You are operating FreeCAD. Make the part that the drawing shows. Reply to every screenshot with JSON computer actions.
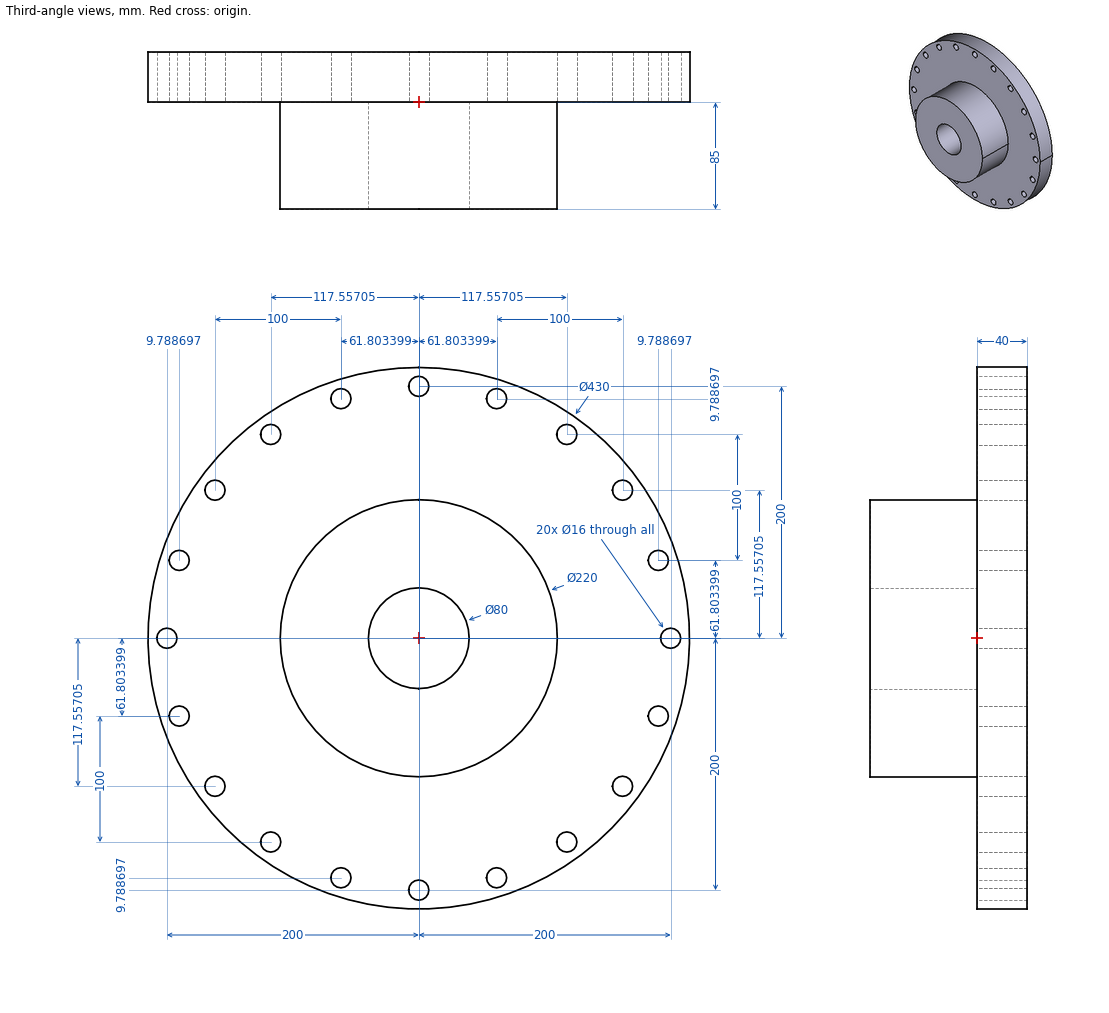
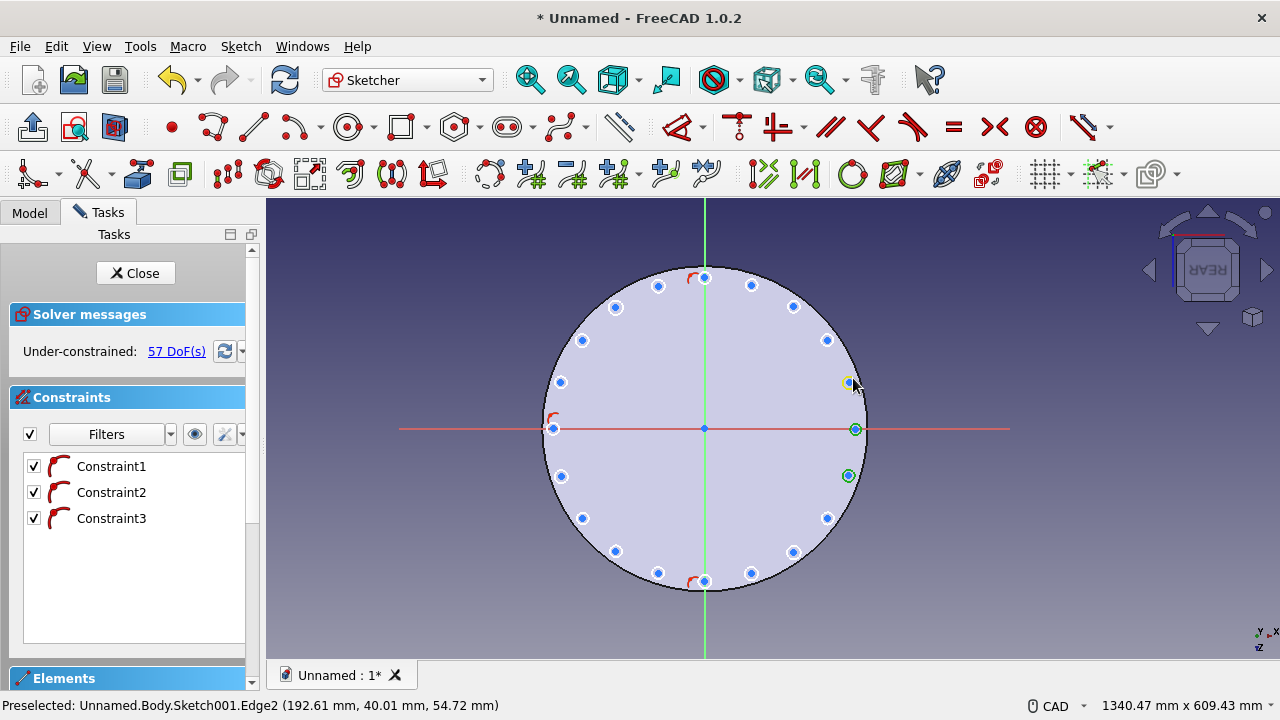
{"action": "scroll", "coordinate": [832, 514], "scroll_direction": "up", "scroll_amount": 5}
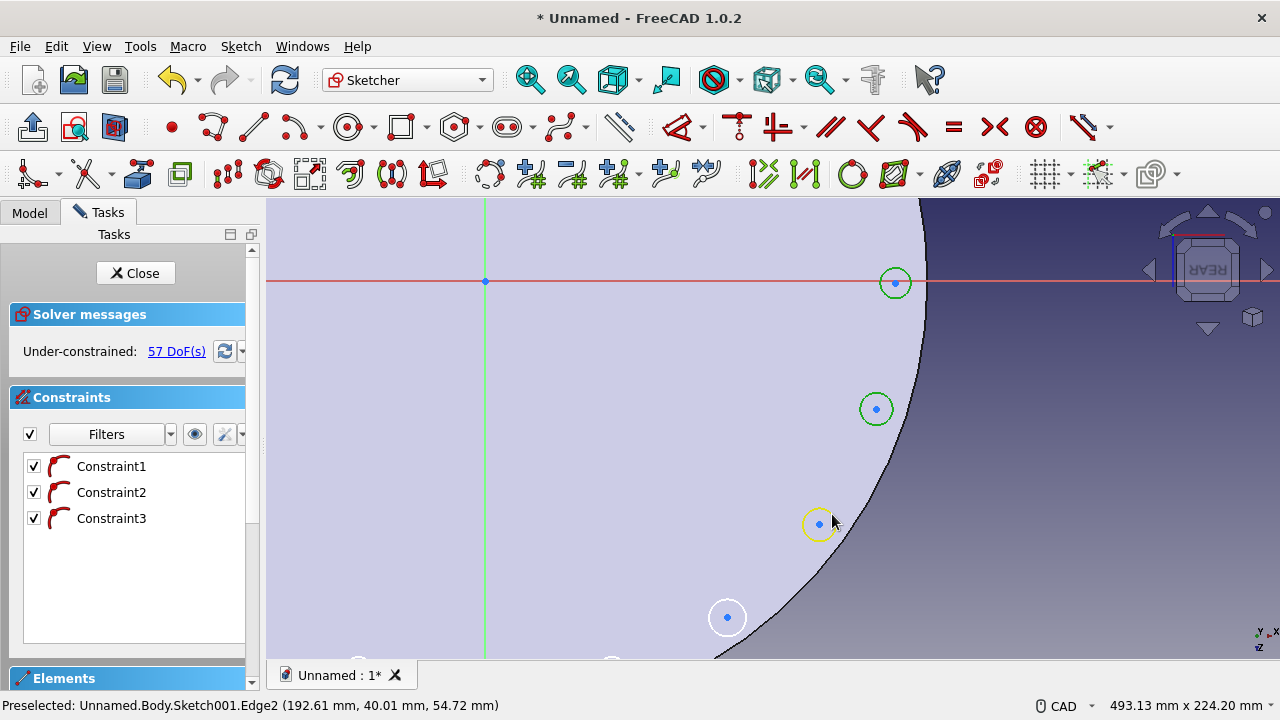
{"action": "left_click", "coordinate": [831, 513]}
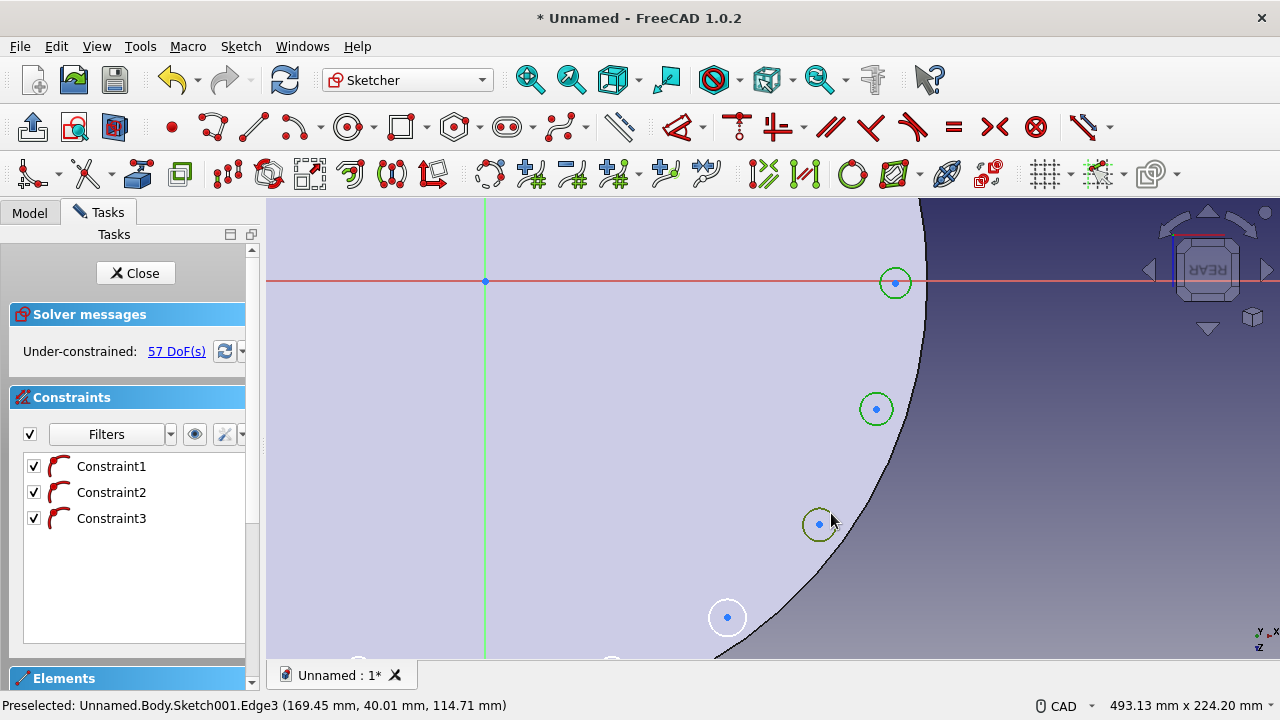
{"action": "left_click", "coordinate": [741, 605]}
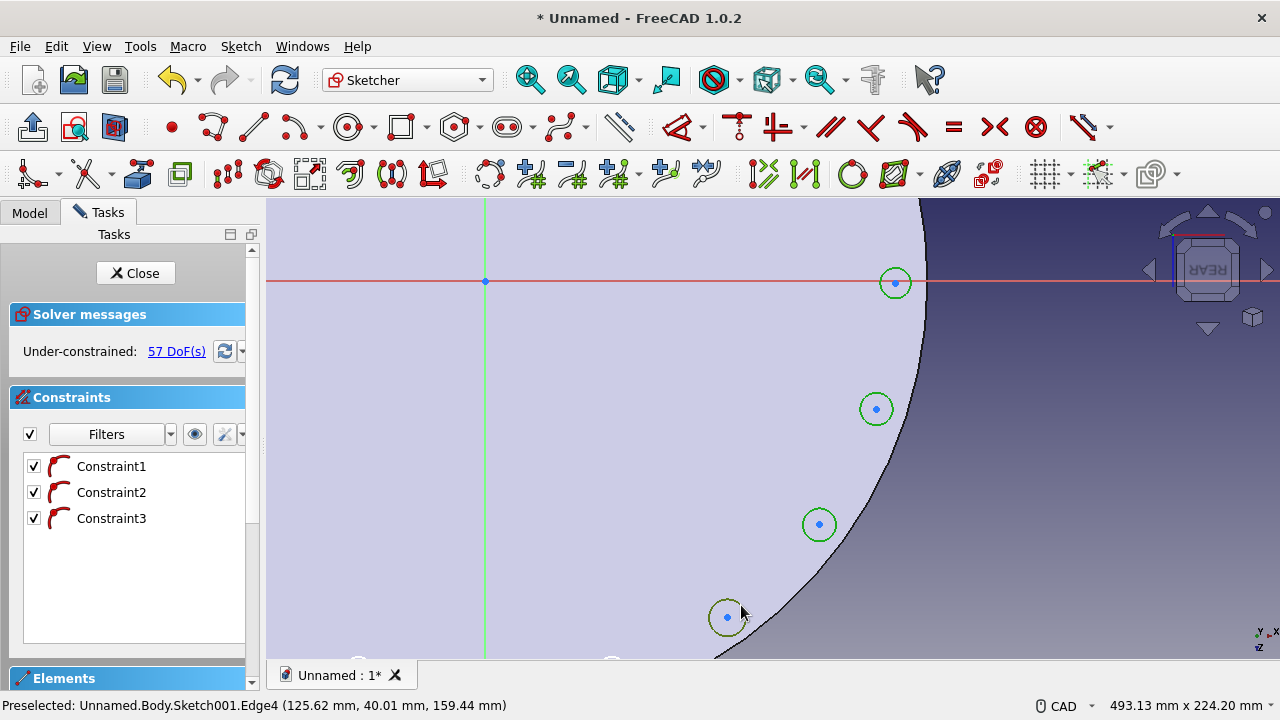
{"action": "scroll", "coordinate": [832, 514], "scroll_direction": "down", "scroll_amount": 5}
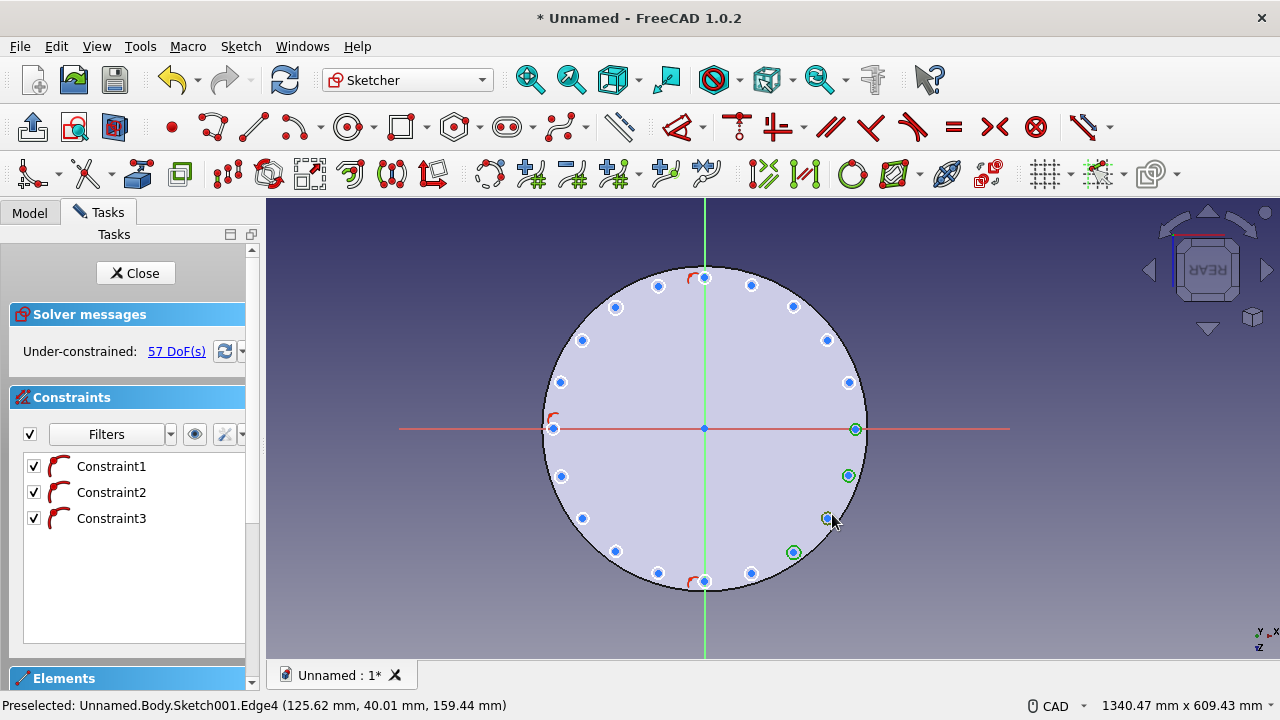
{"action": "scroll", "coordinate": [756, 569], "scroll_direction": "up", "scroll_amount": 4}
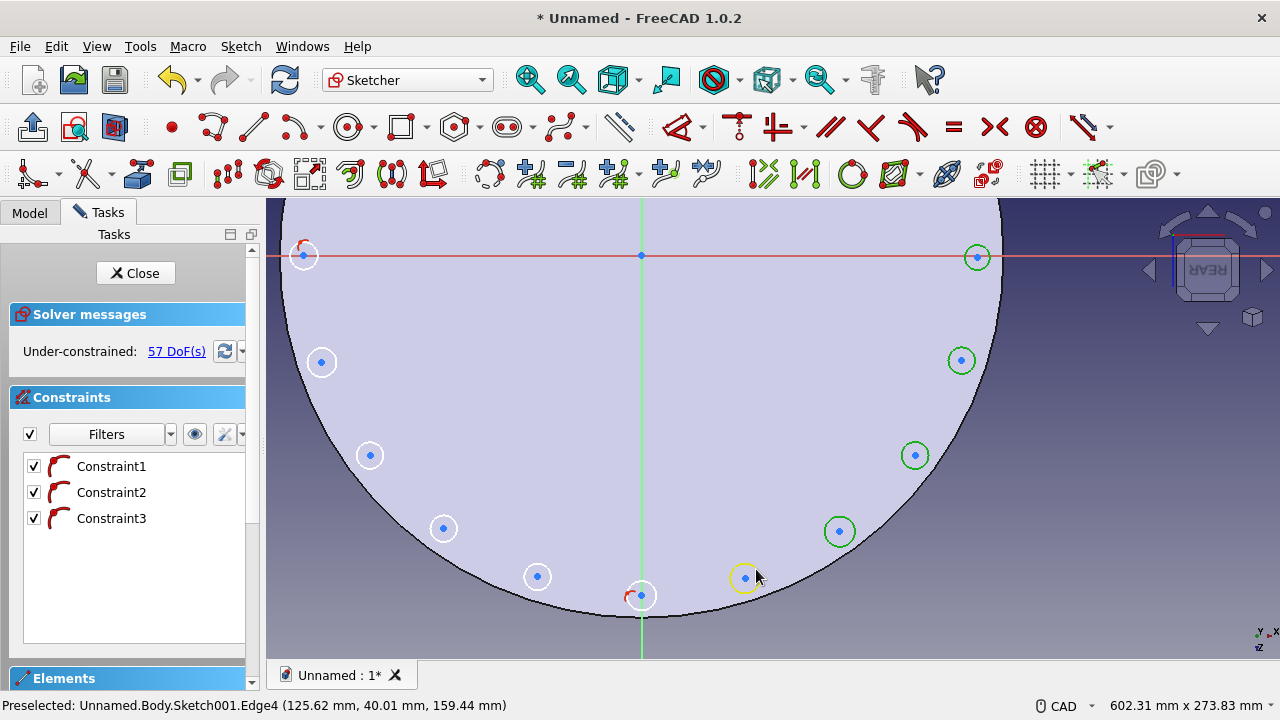
{"action": "left_click", "coordinate": [756, 568]}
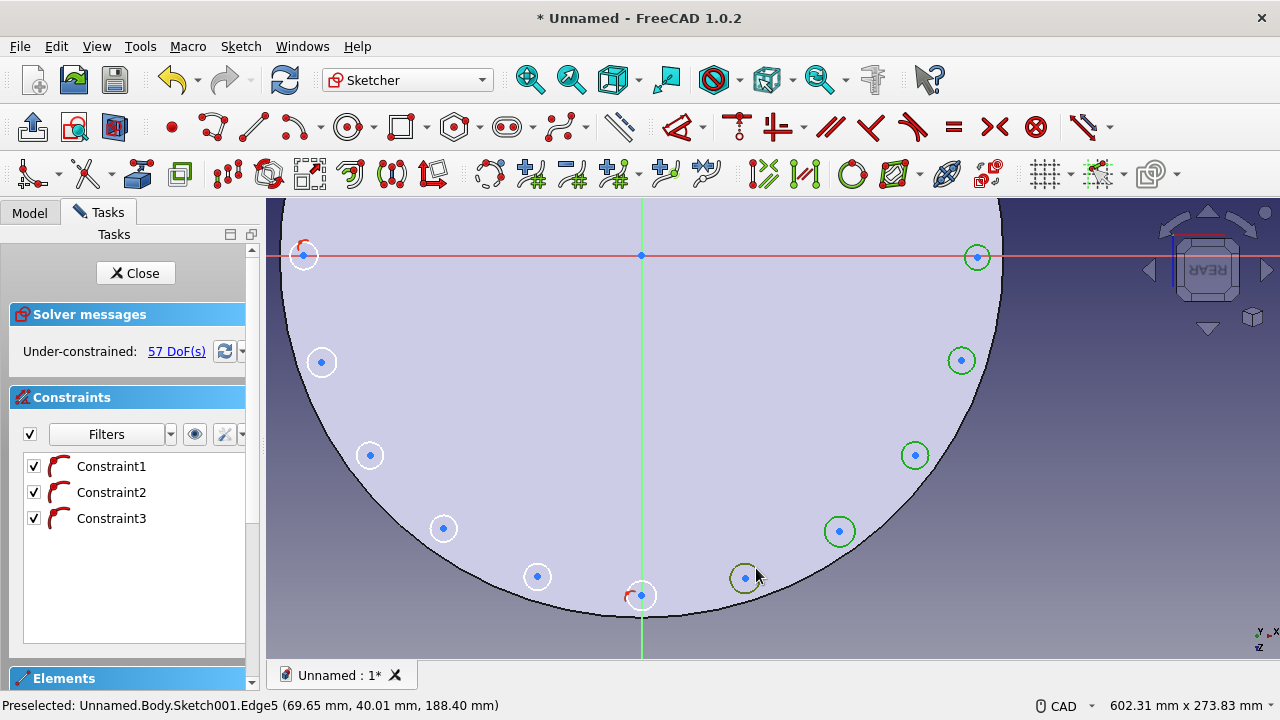
{"action": "scroll", "coordinate": [652, 585], "scroll_direction": "up", "scroll_amount": 2}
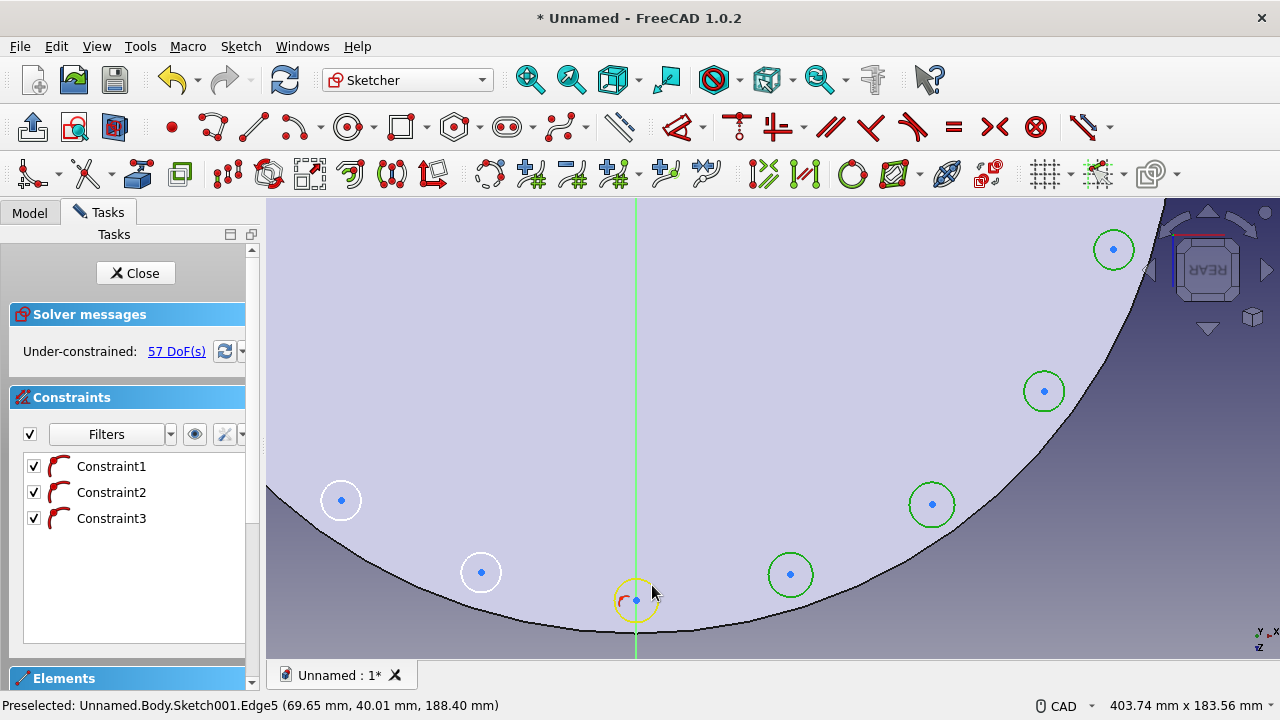
{"action": "left_click", "coordinate": [652, 585]}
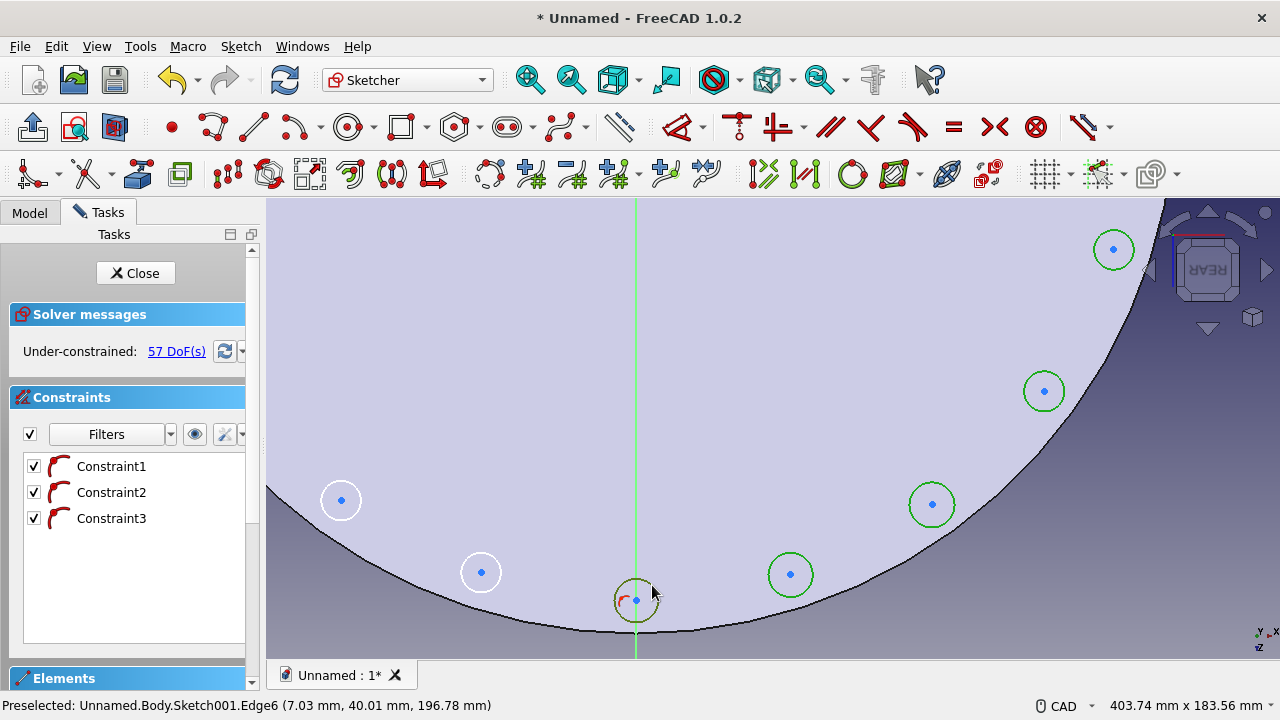
{"action": "left_click", "coordinate": [495, 559]}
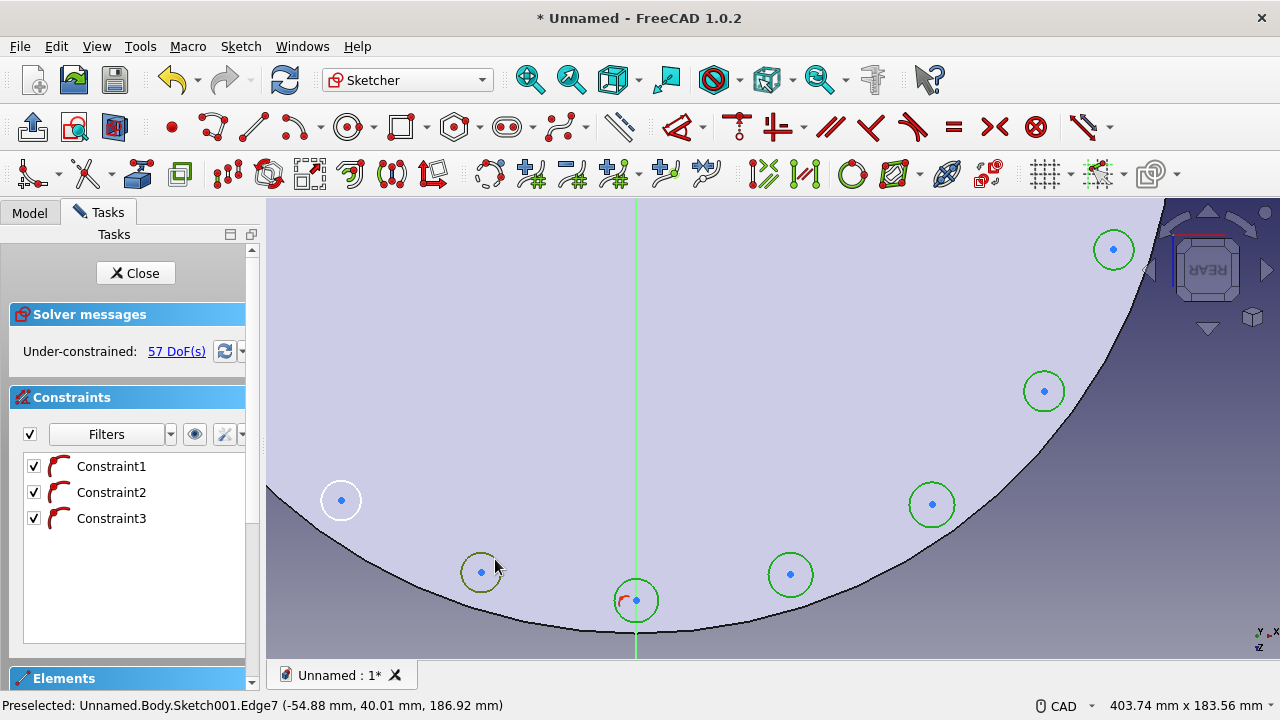
{"action": "left_click", "coordinate": [355, 487]}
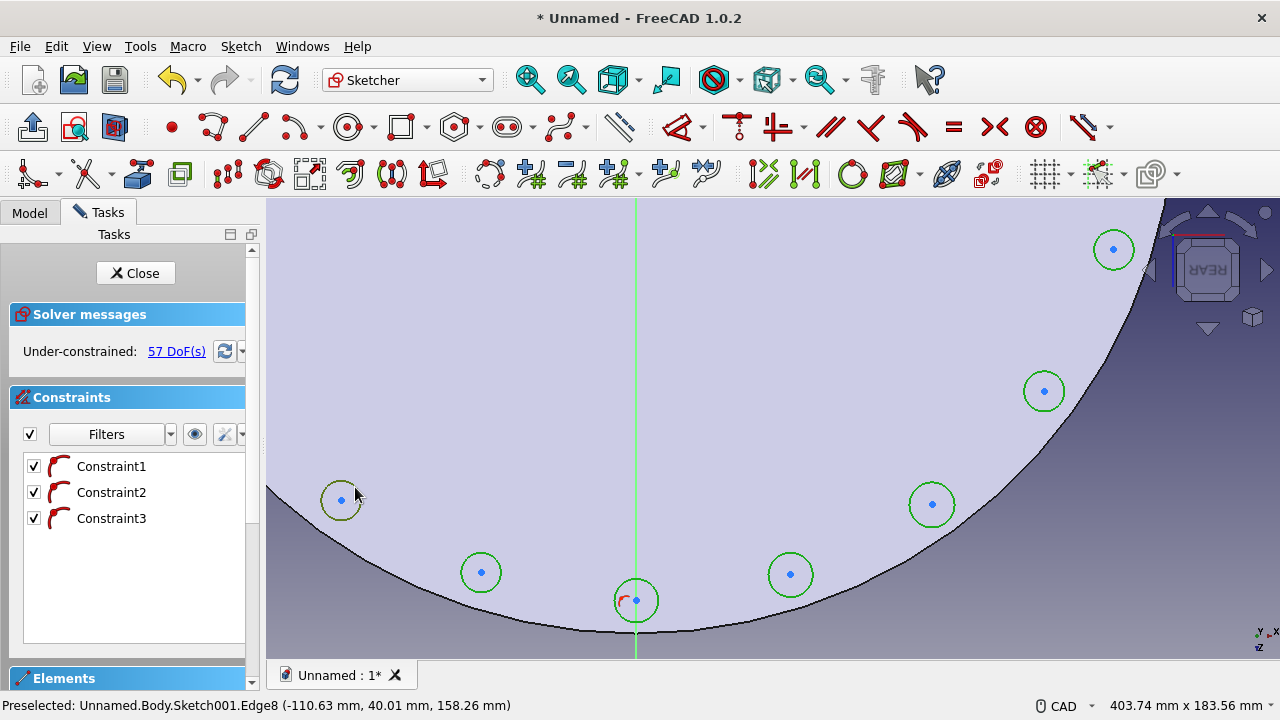
{"action": "scroll", "coordinate": [734, 573], "scroll_direction": "down", "scroll_amount": 6}